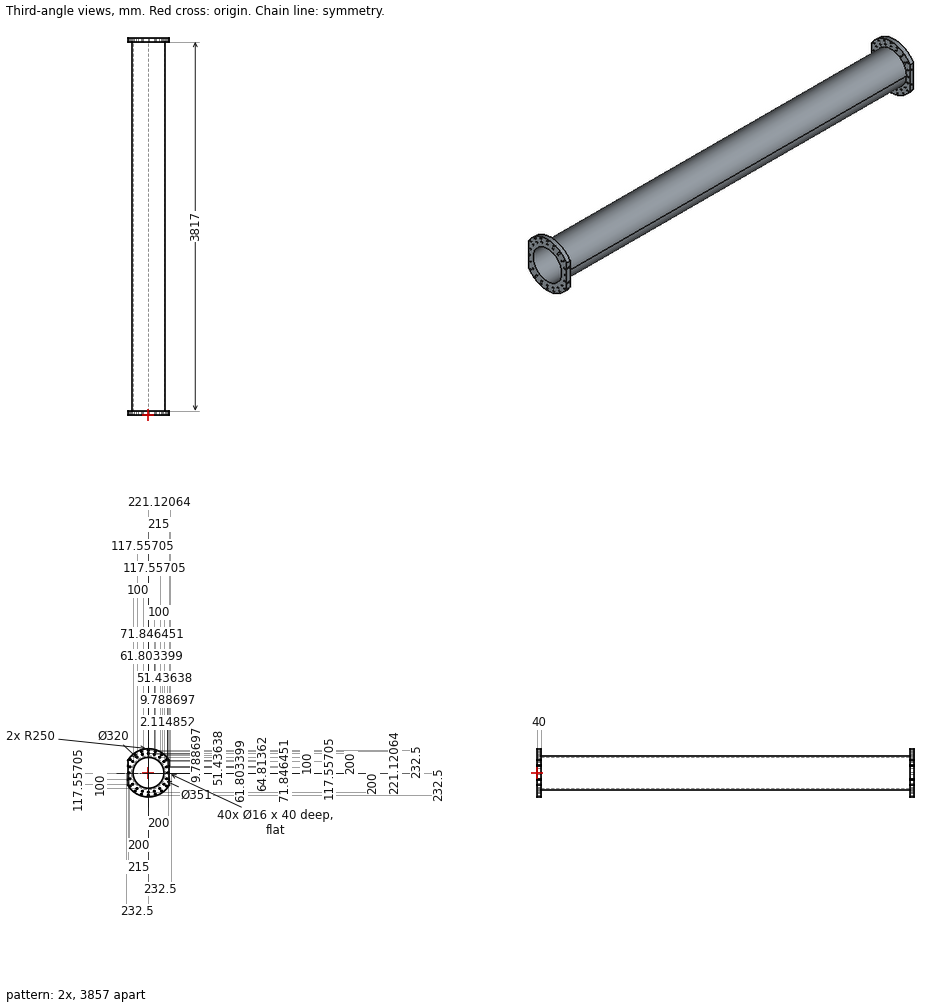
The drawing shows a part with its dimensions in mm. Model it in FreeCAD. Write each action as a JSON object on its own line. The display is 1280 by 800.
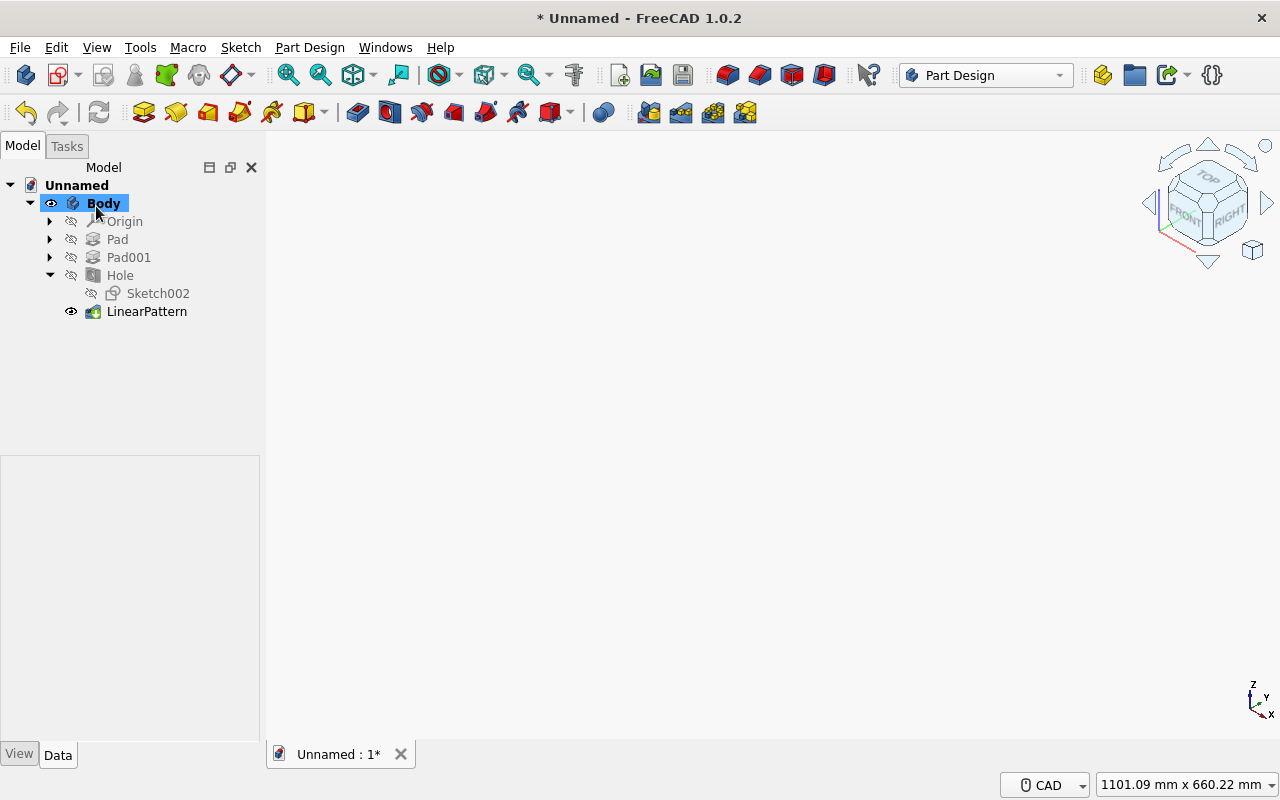
{"action": "left_click", "coordinate": [290, 76]}